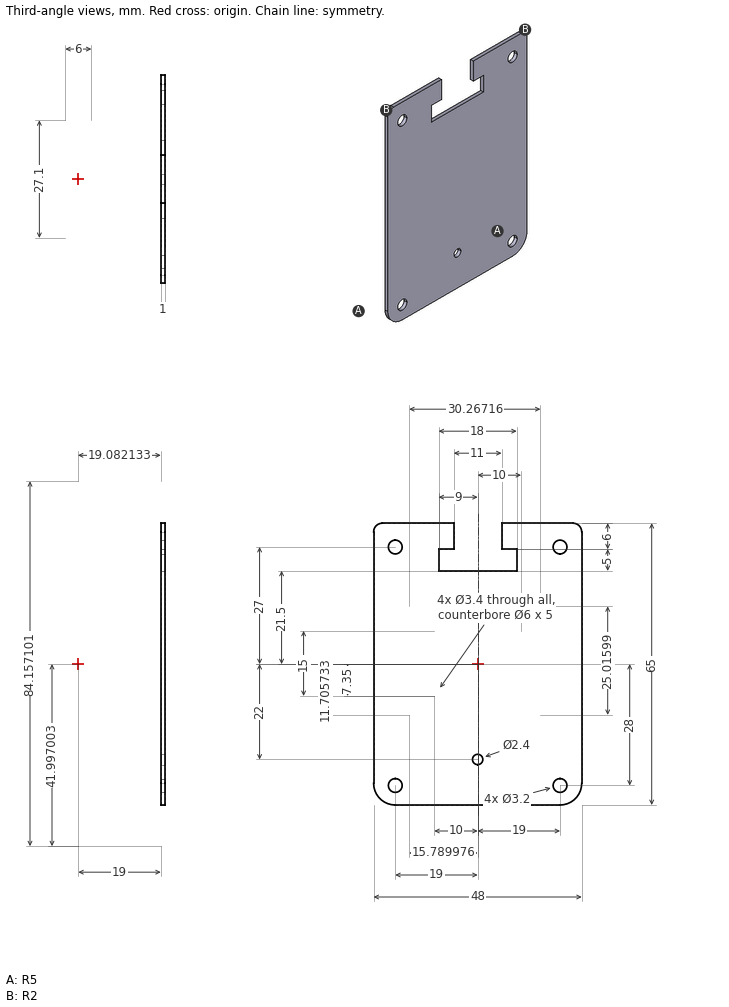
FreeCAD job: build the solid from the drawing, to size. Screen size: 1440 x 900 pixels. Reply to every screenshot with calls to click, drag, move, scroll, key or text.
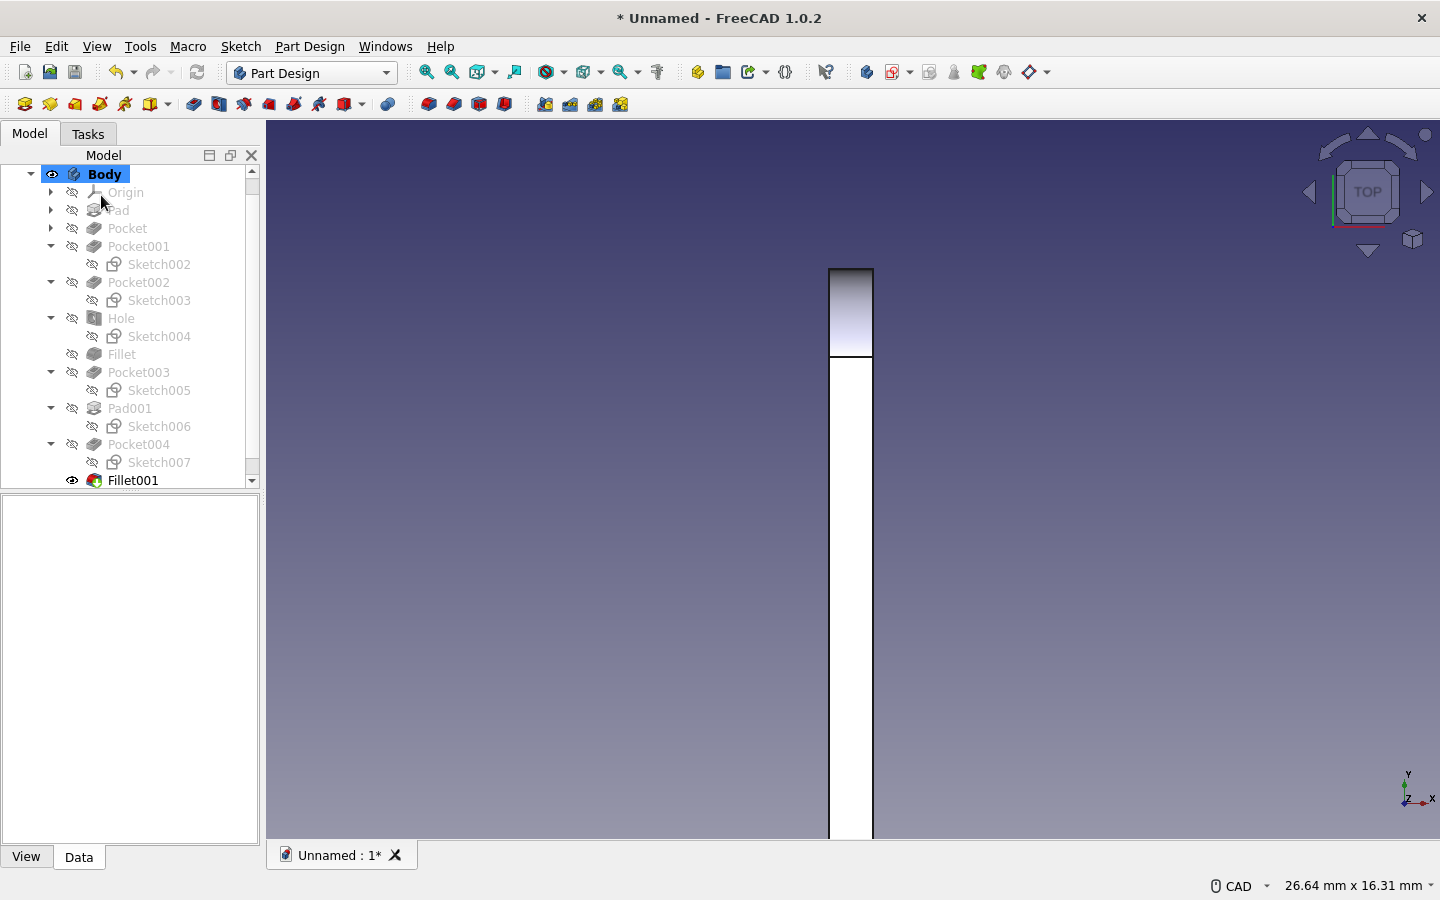
key(0)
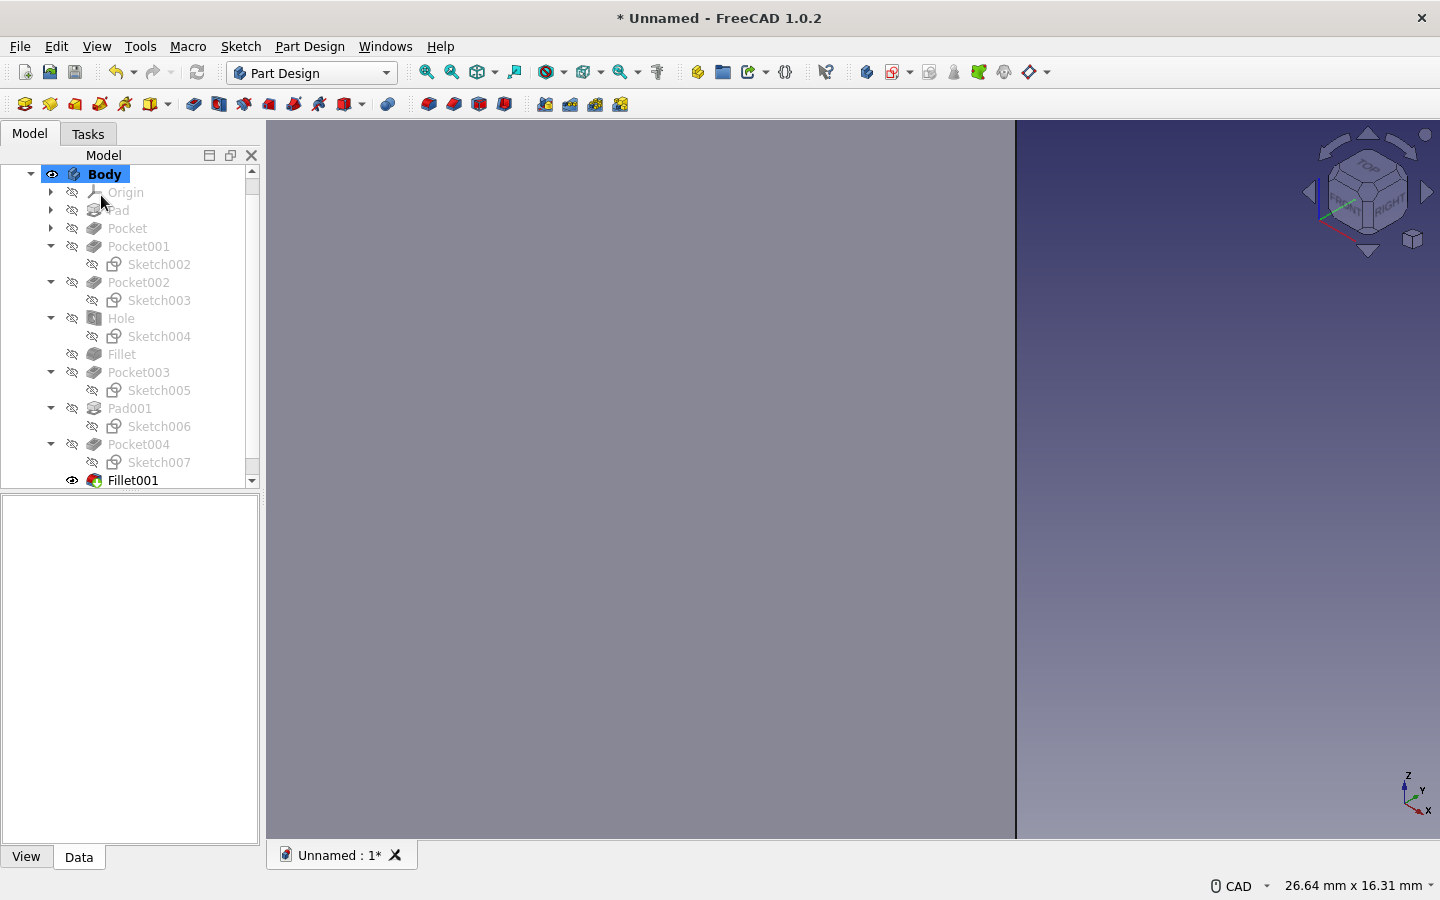
key(v)
key(f)